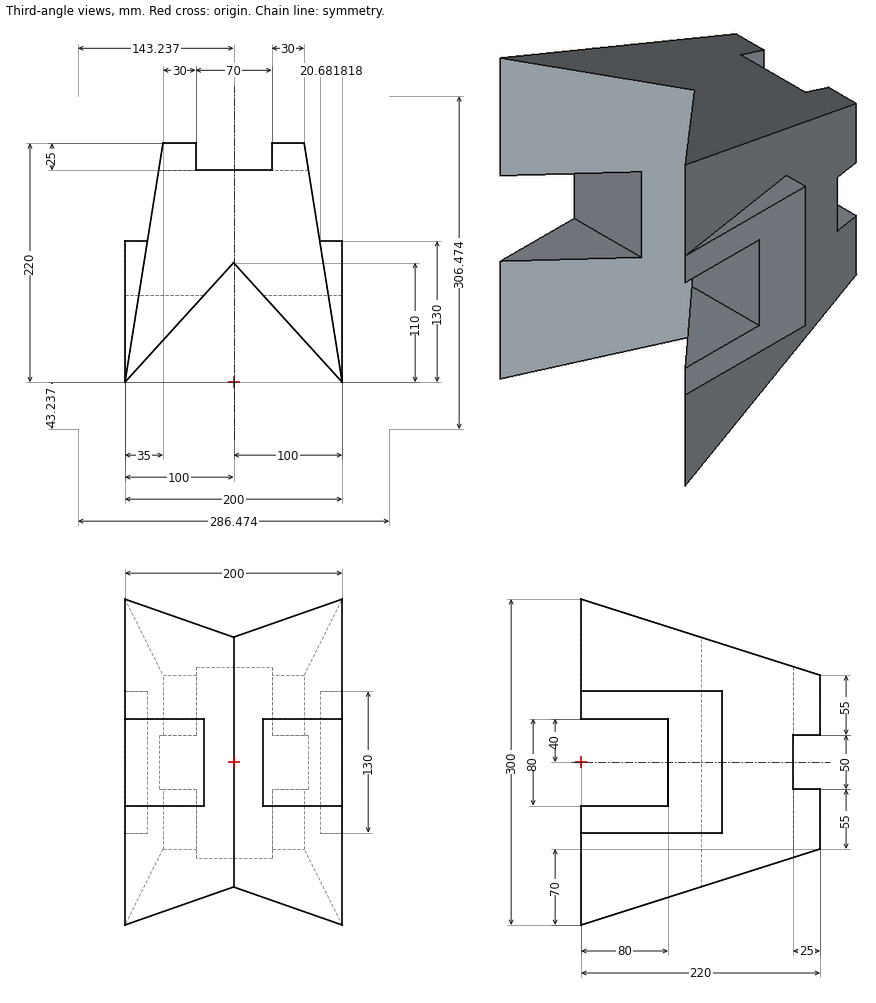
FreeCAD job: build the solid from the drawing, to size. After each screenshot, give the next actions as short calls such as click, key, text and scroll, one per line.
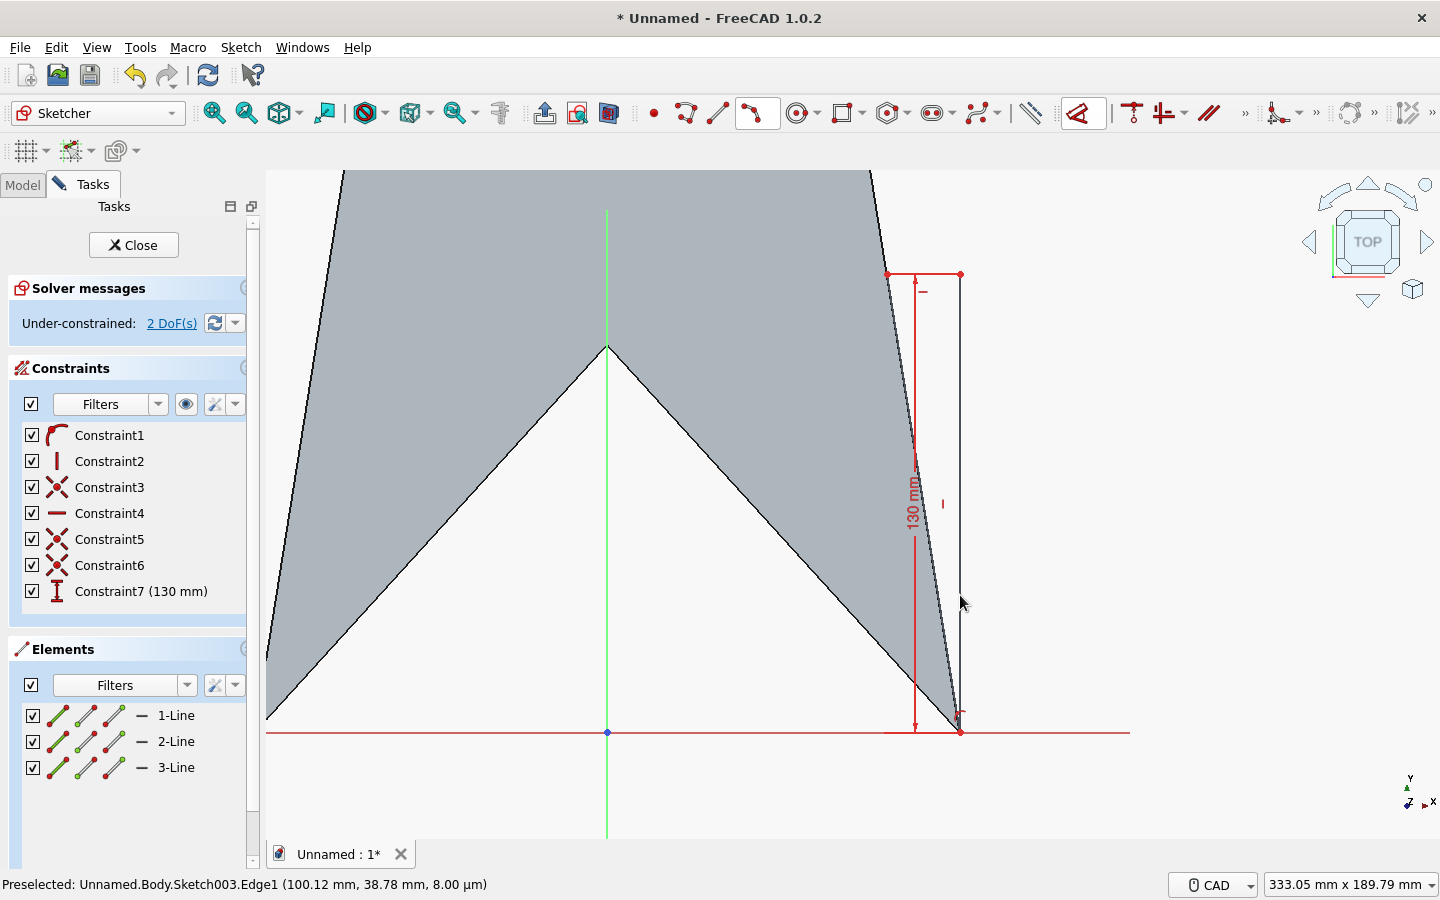
click(960, 733)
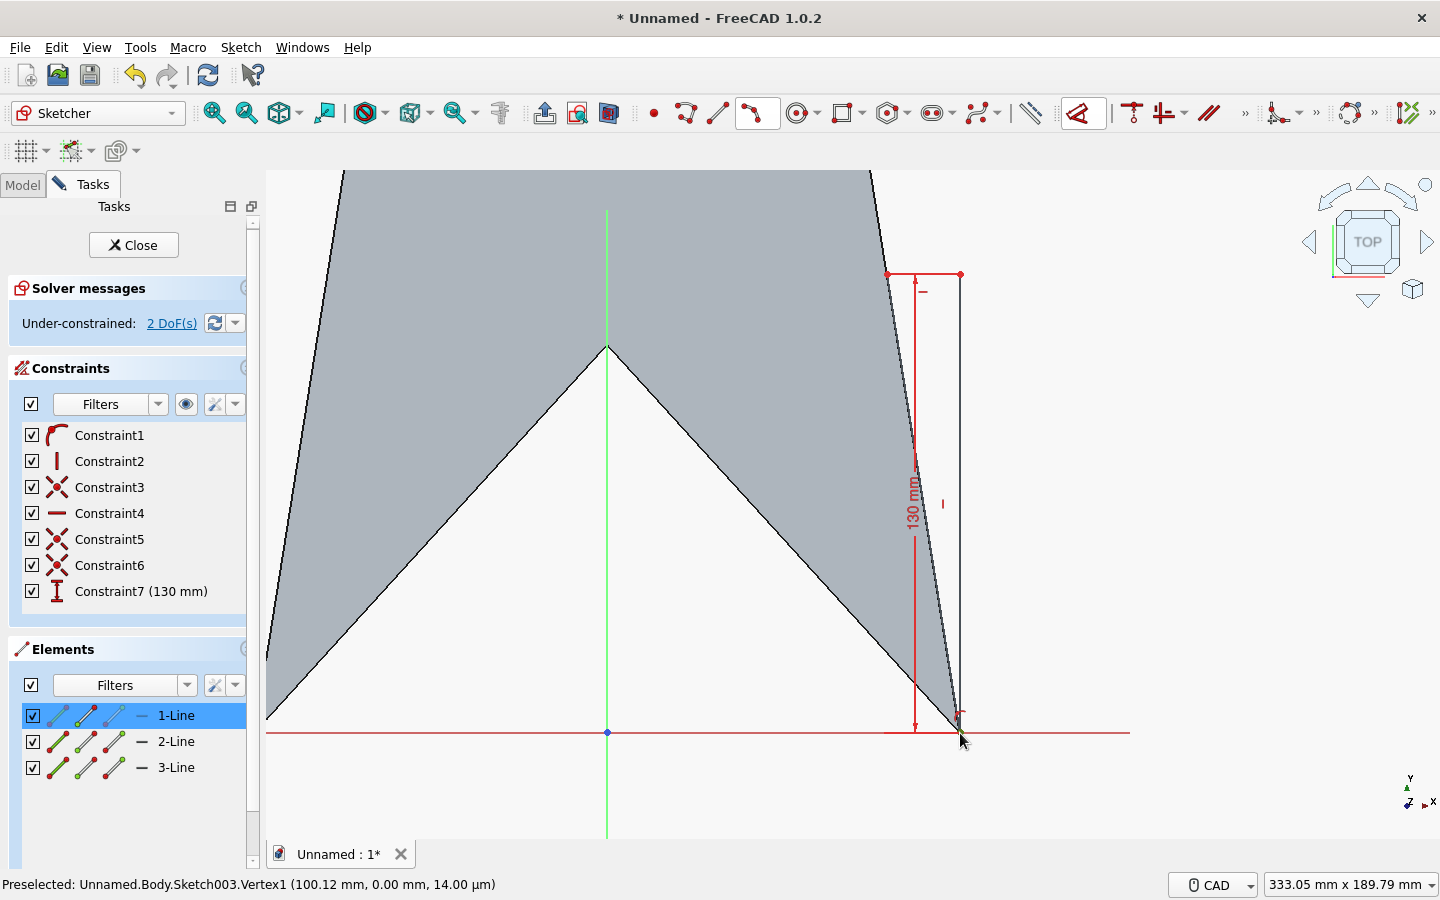
click(1100, 114)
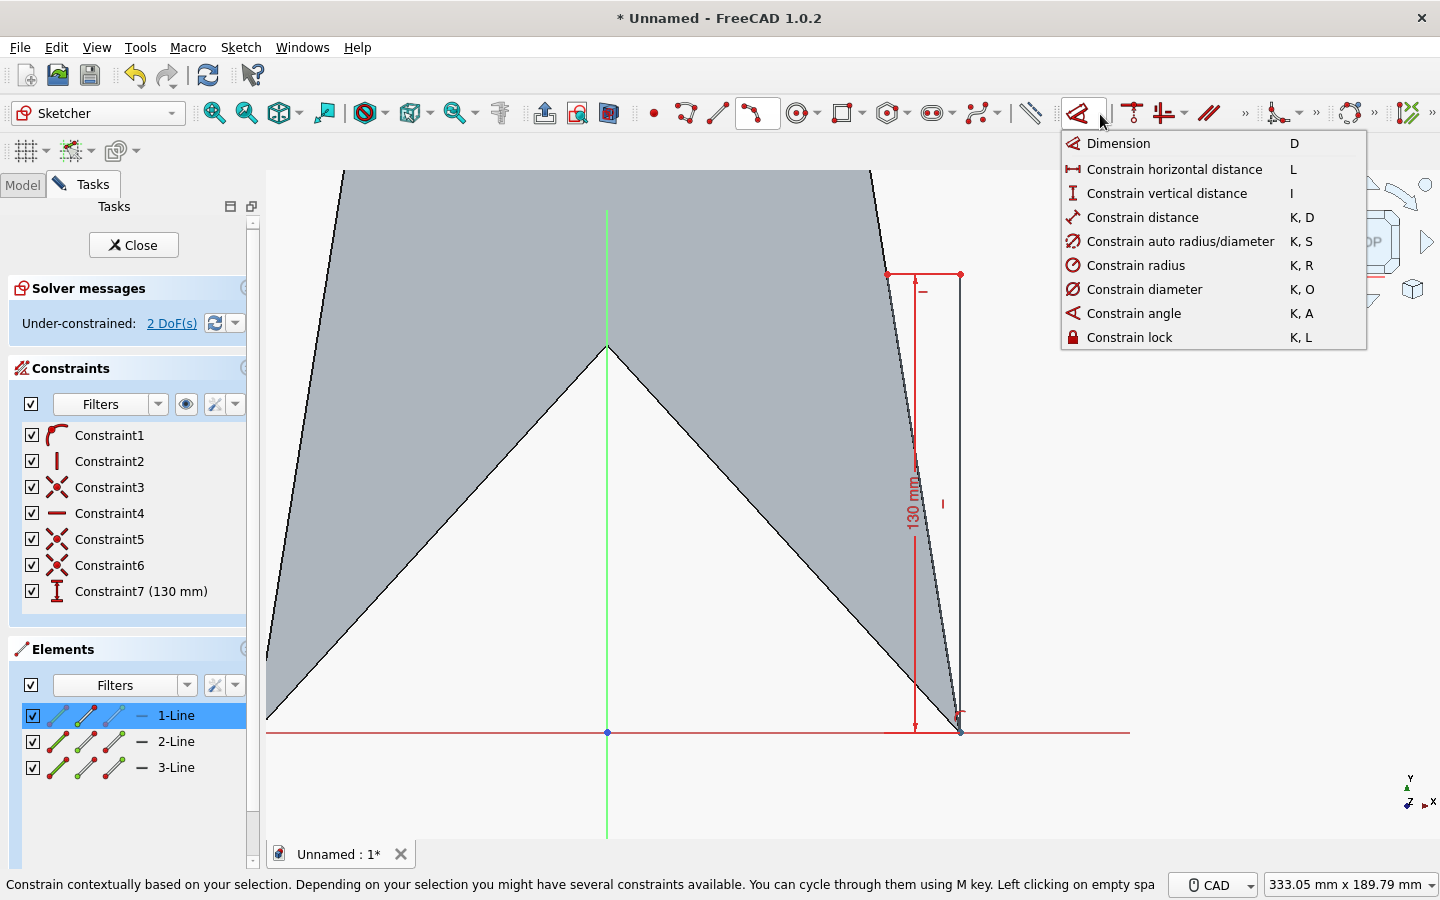
click(1214, 169)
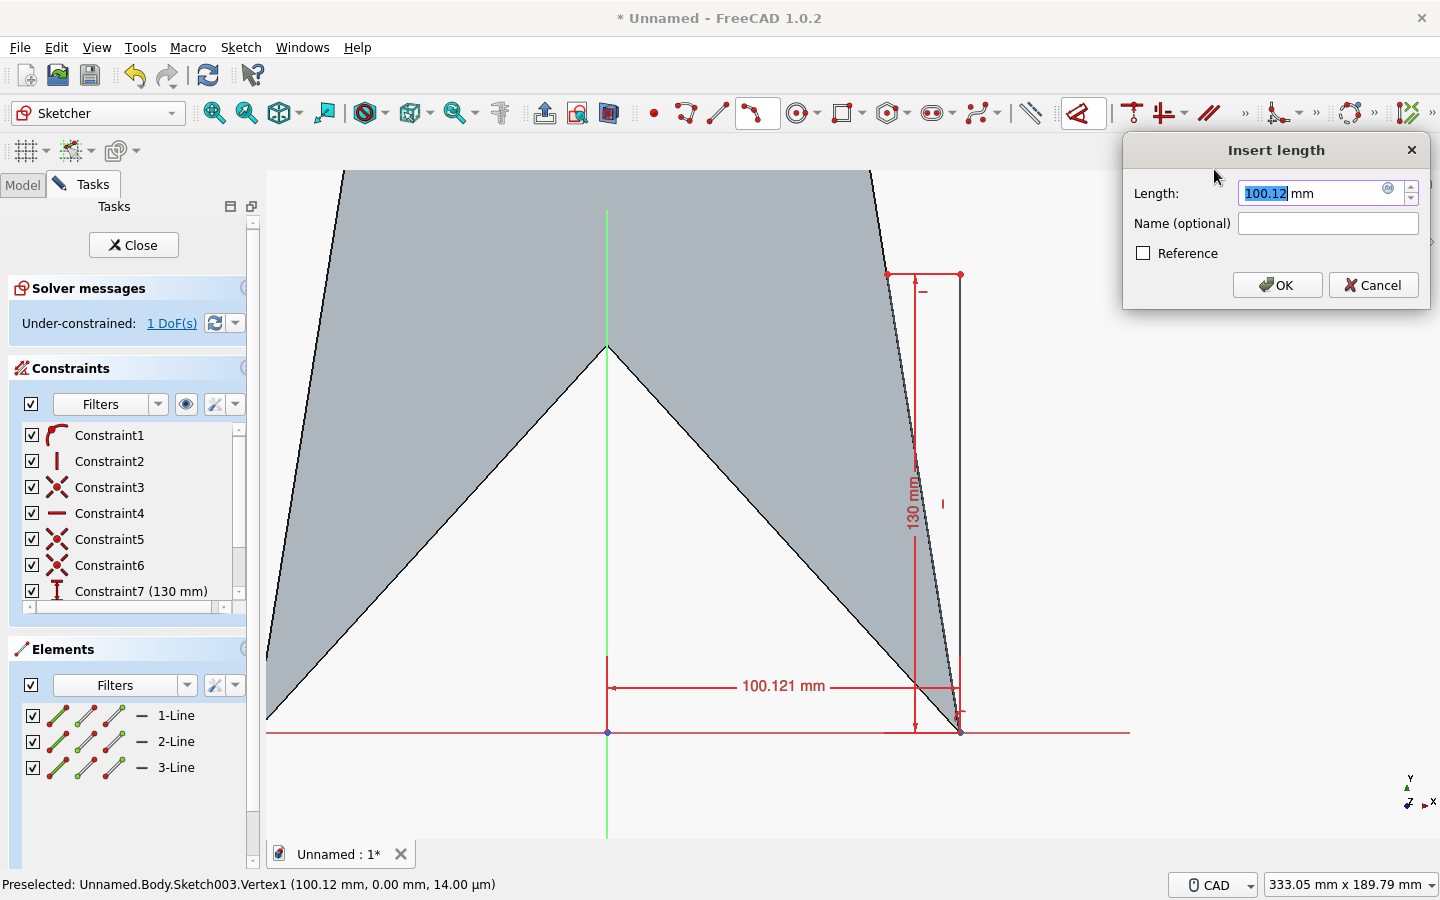
text(100)
key(Return)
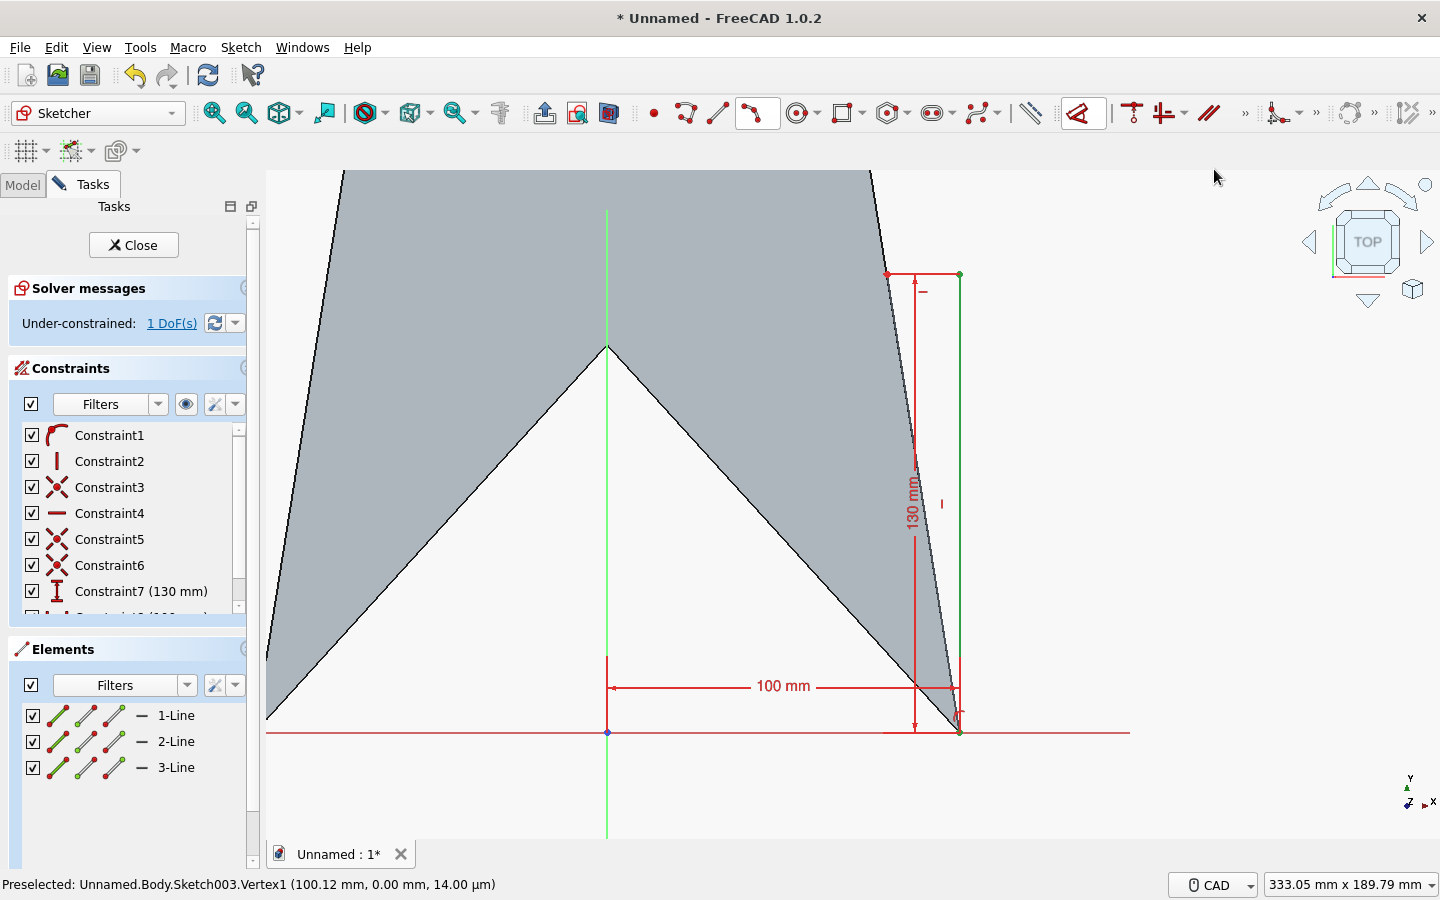
click(938, 274)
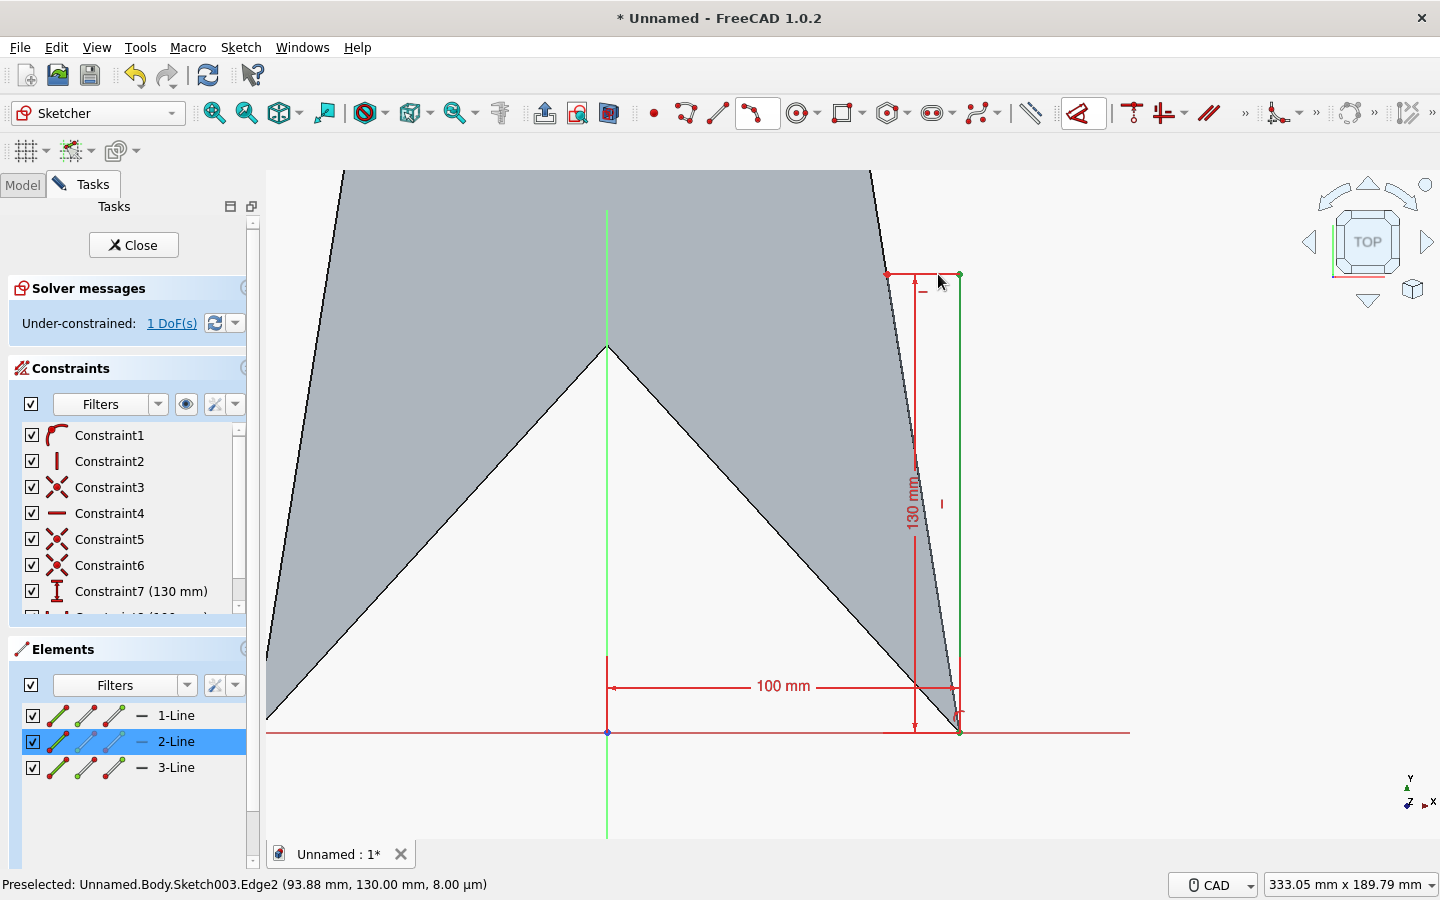
key(l)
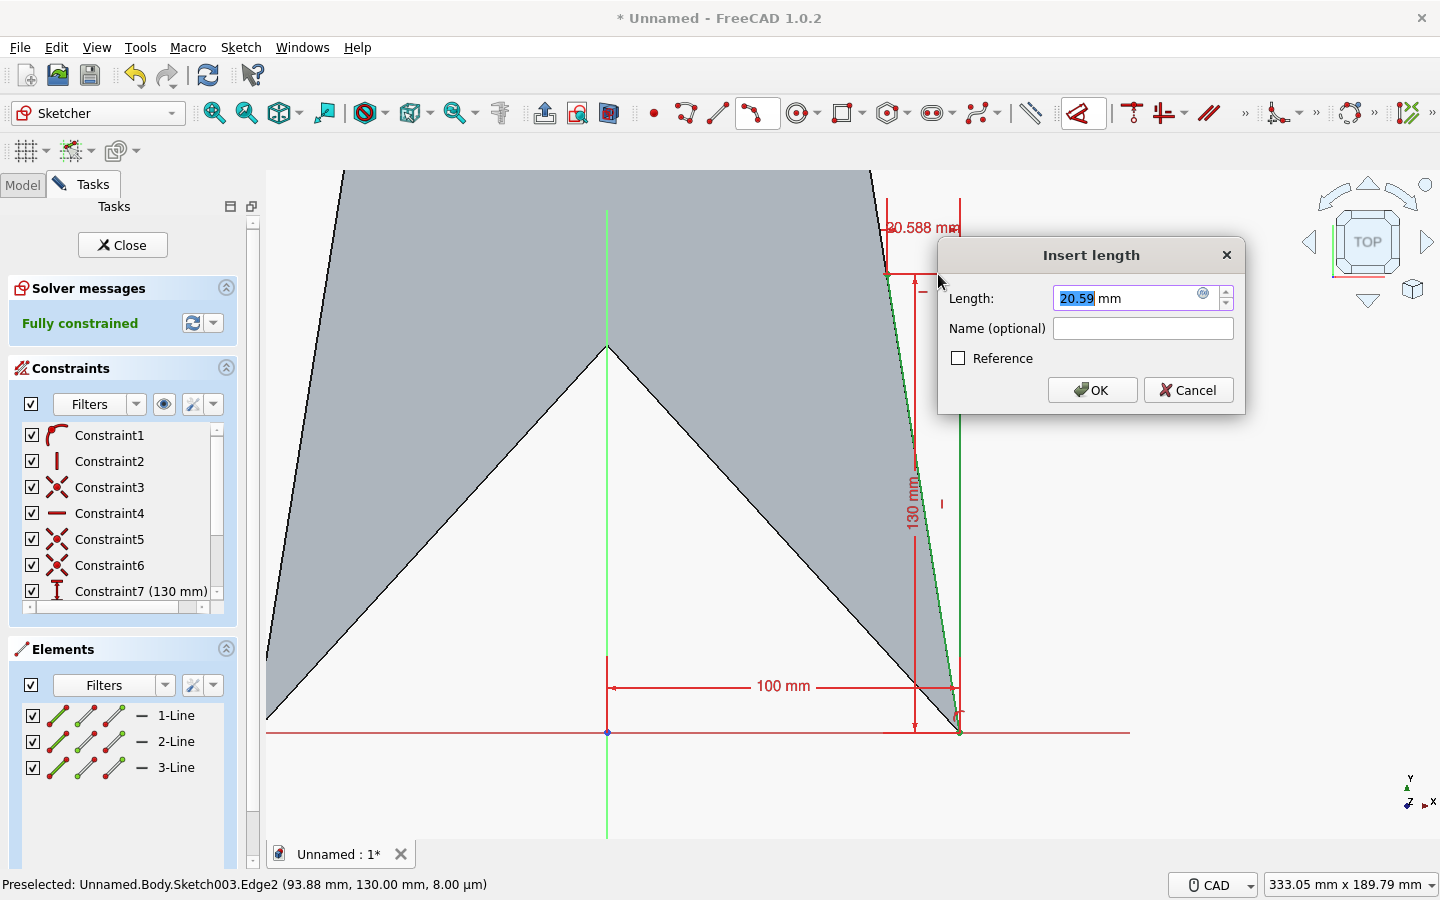
text(20.681818)
key(Return)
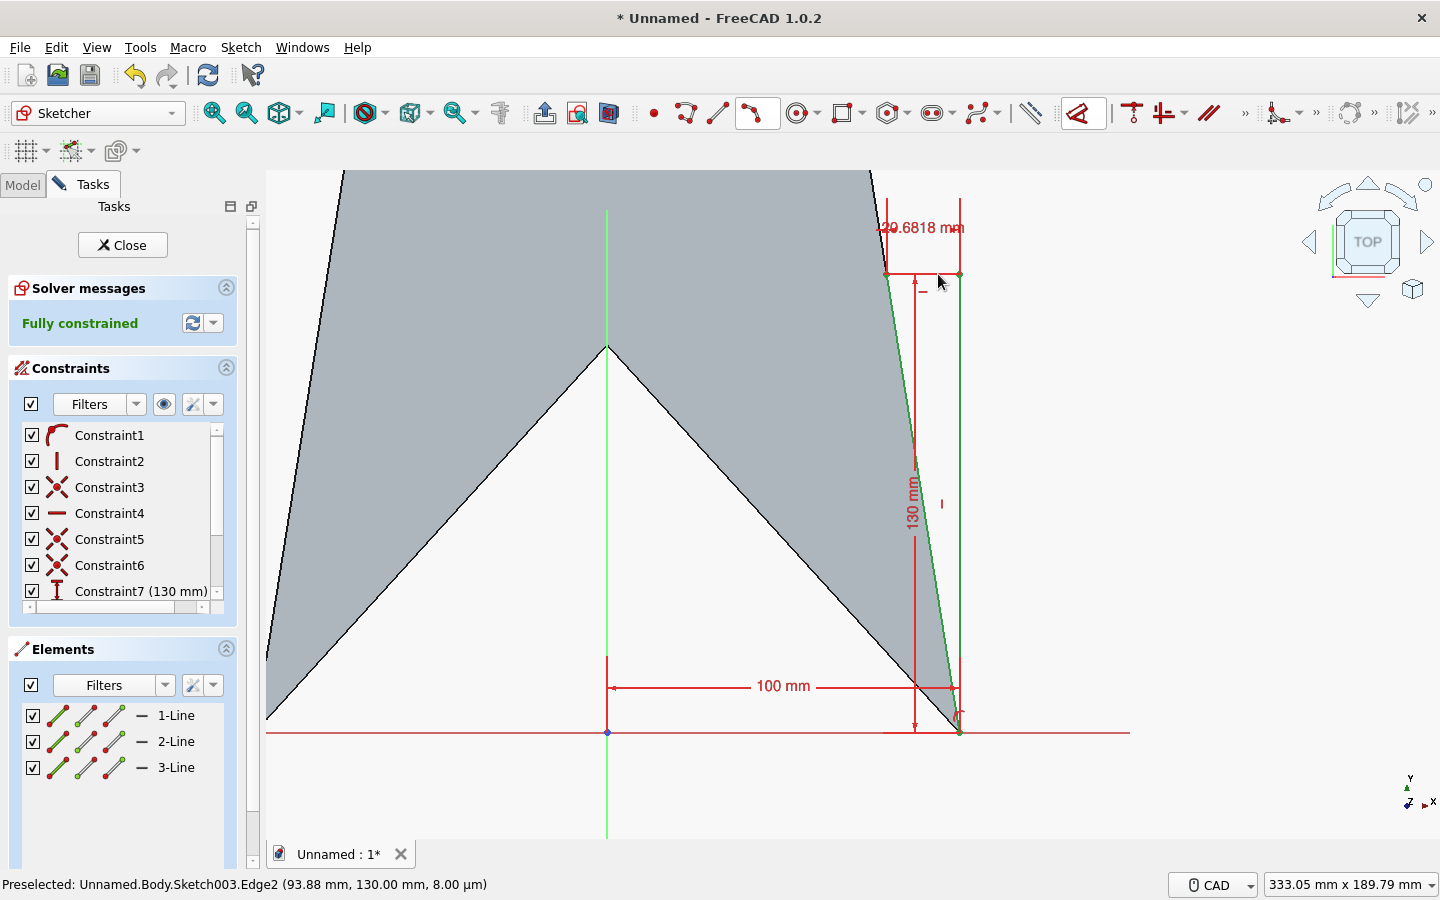
click(123, 245)